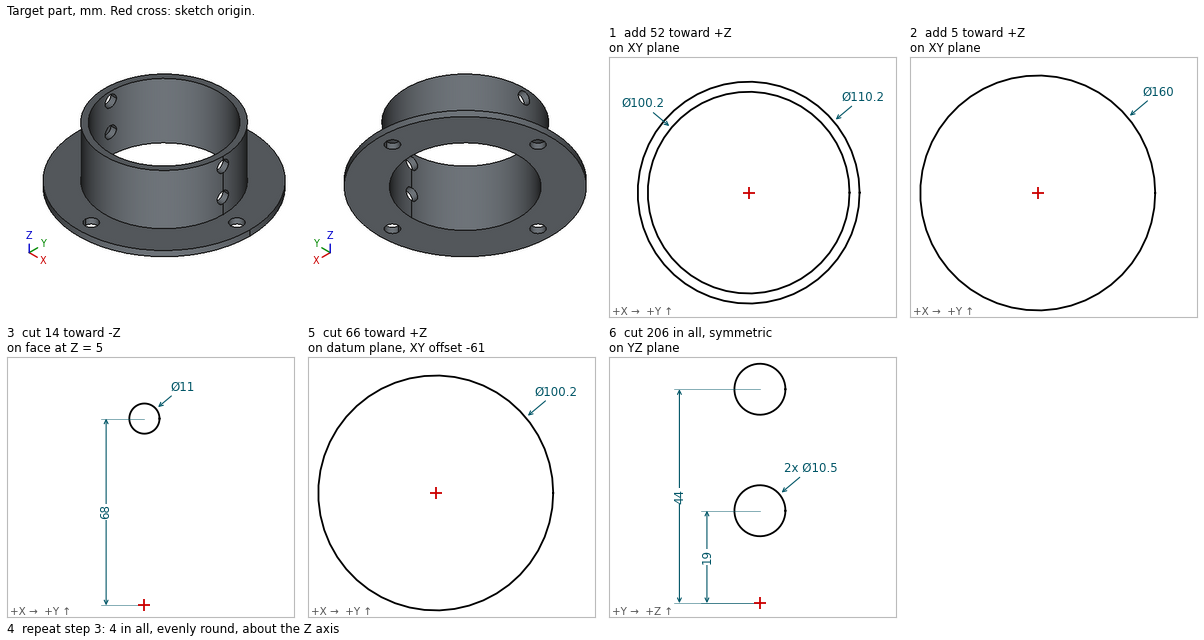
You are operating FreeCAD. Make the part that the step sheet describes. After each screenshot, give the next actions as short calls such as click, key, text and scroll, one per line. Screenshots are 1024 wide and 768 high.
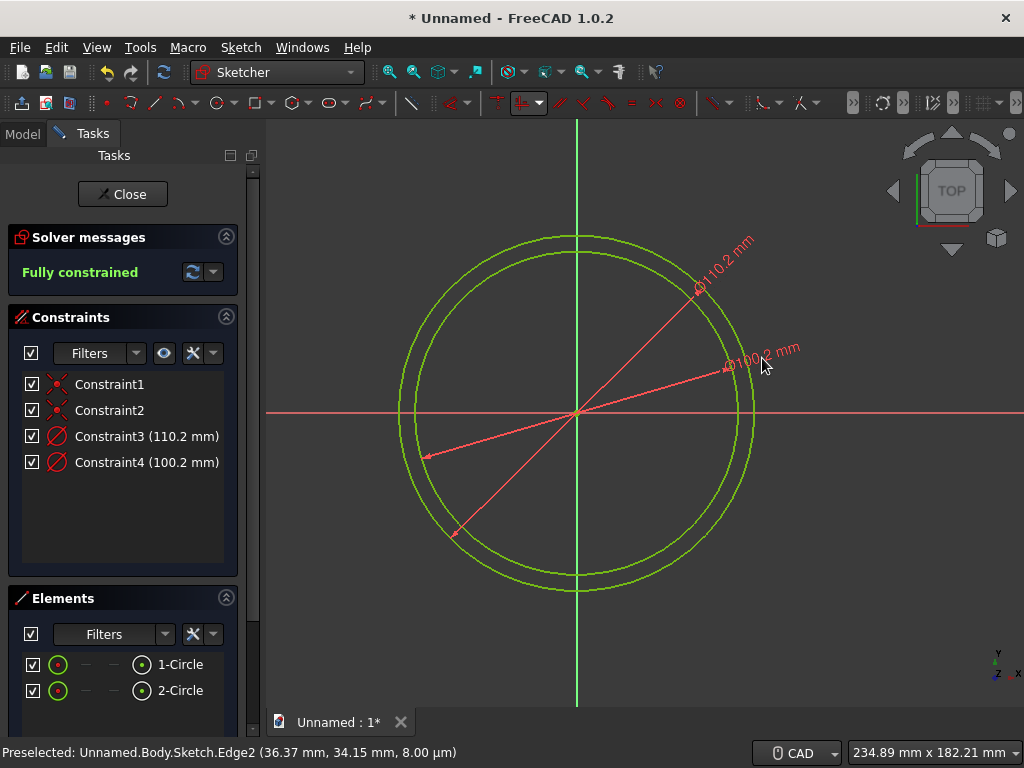
click(123, 194)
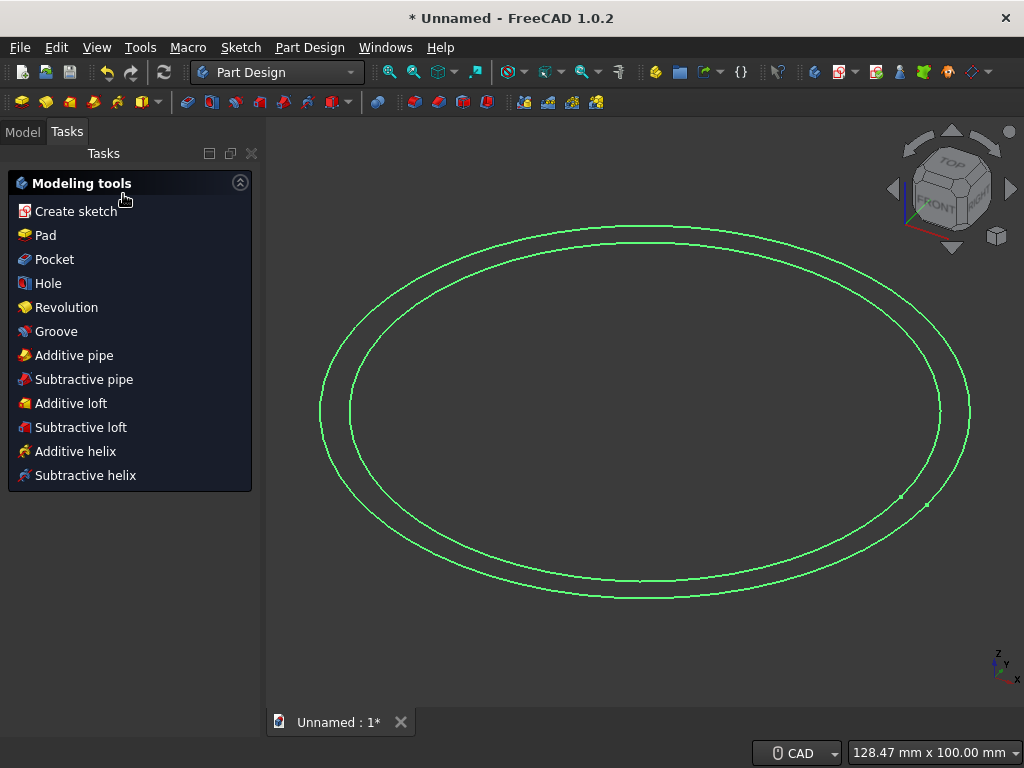
click(22, 102)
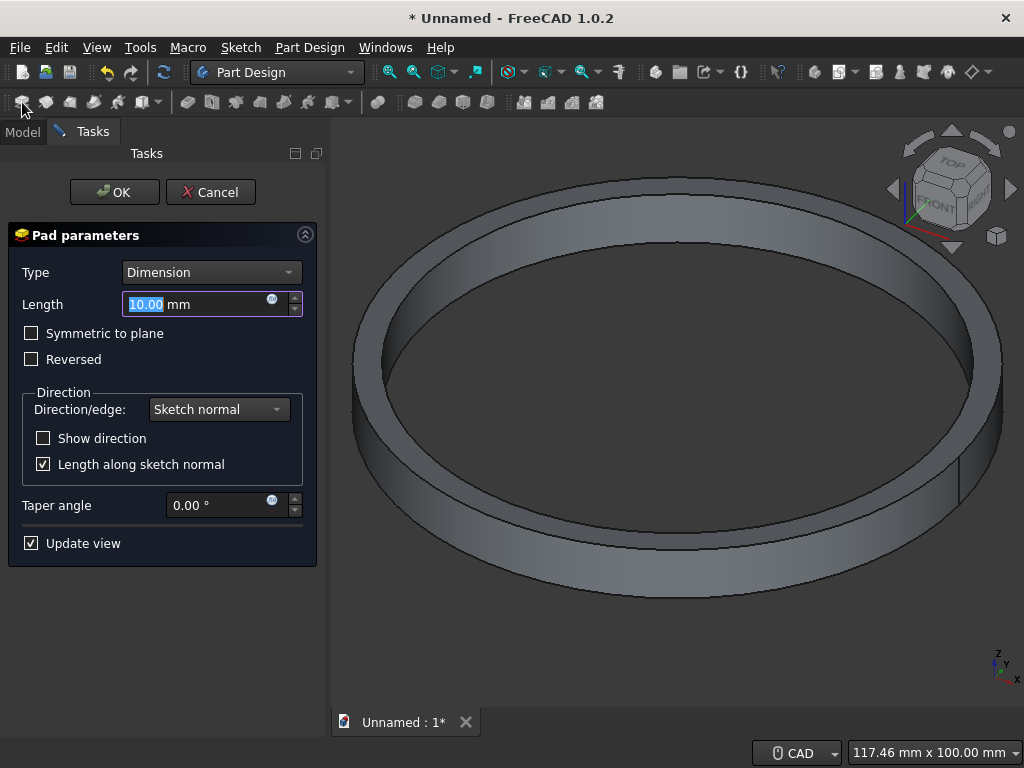
text(52)
key(Tab)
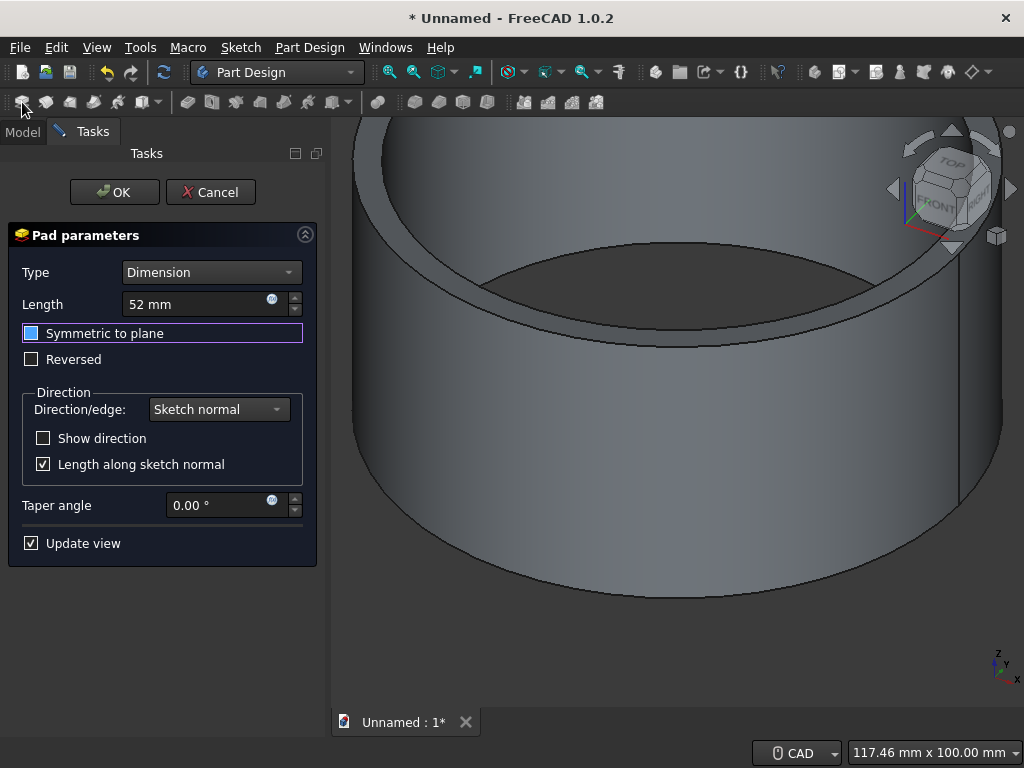
click(115, 192)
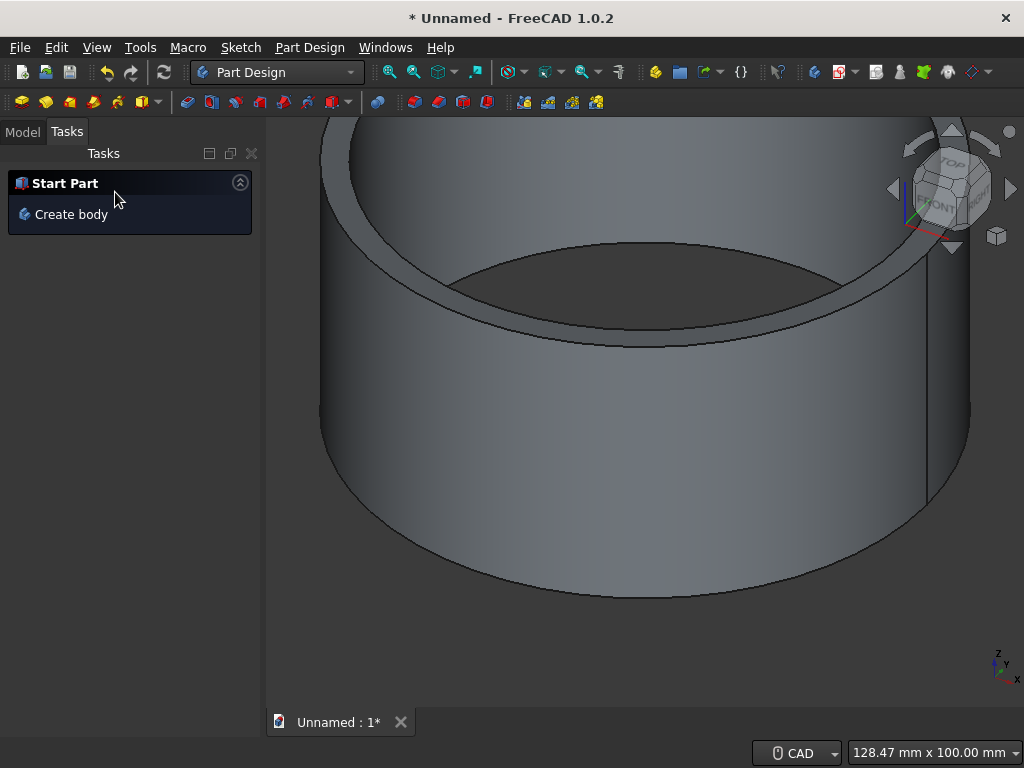
click(390, 72)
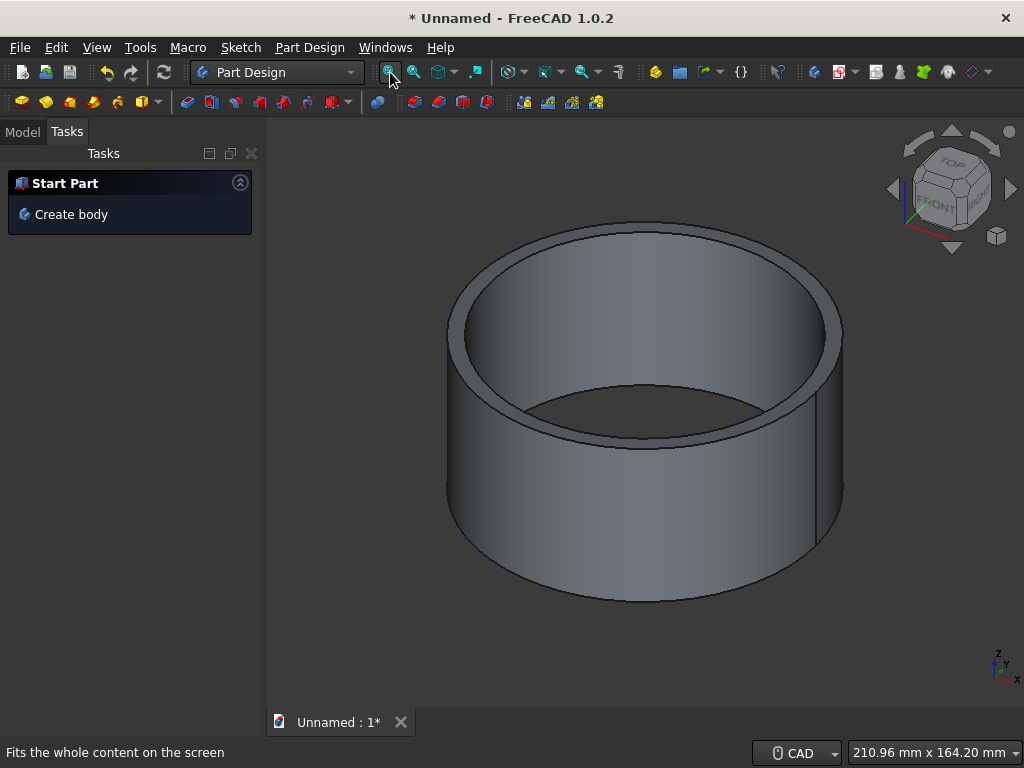
click(840, 72)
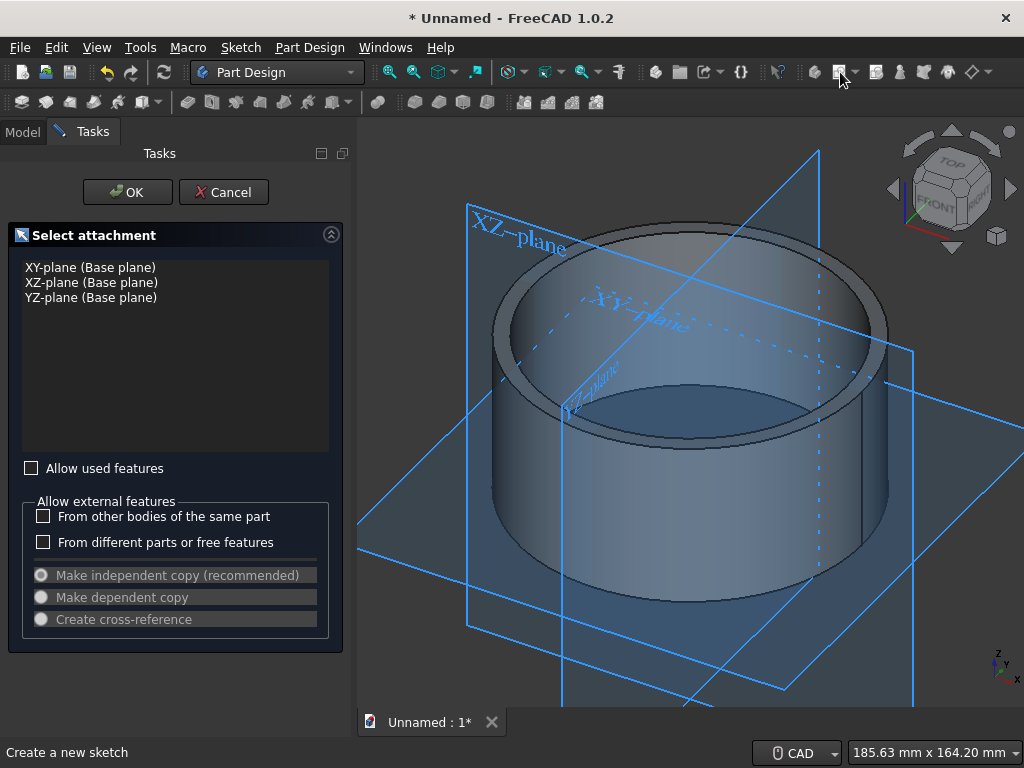
click(82, 268)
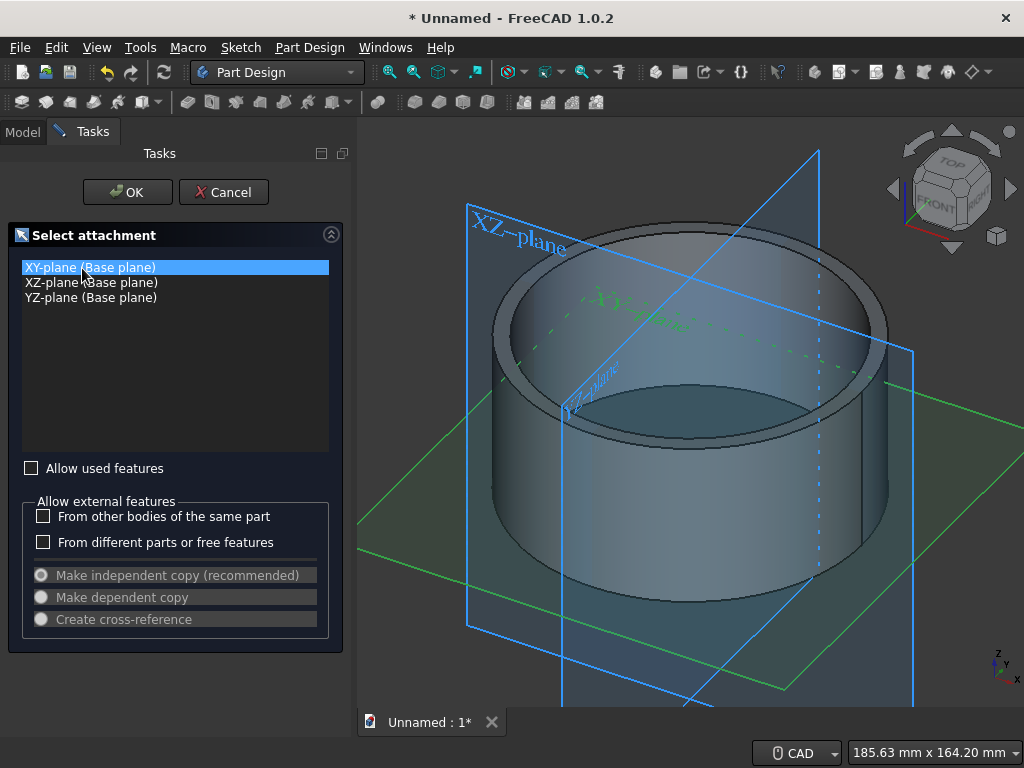
click(128, 192)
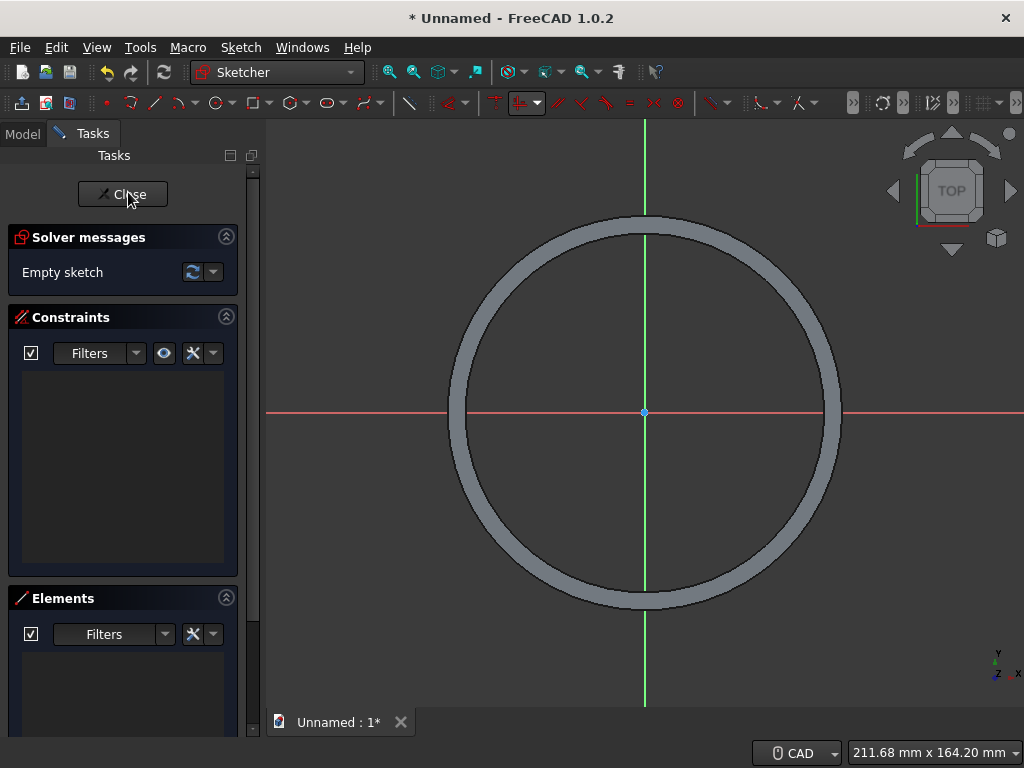
click(70, 104)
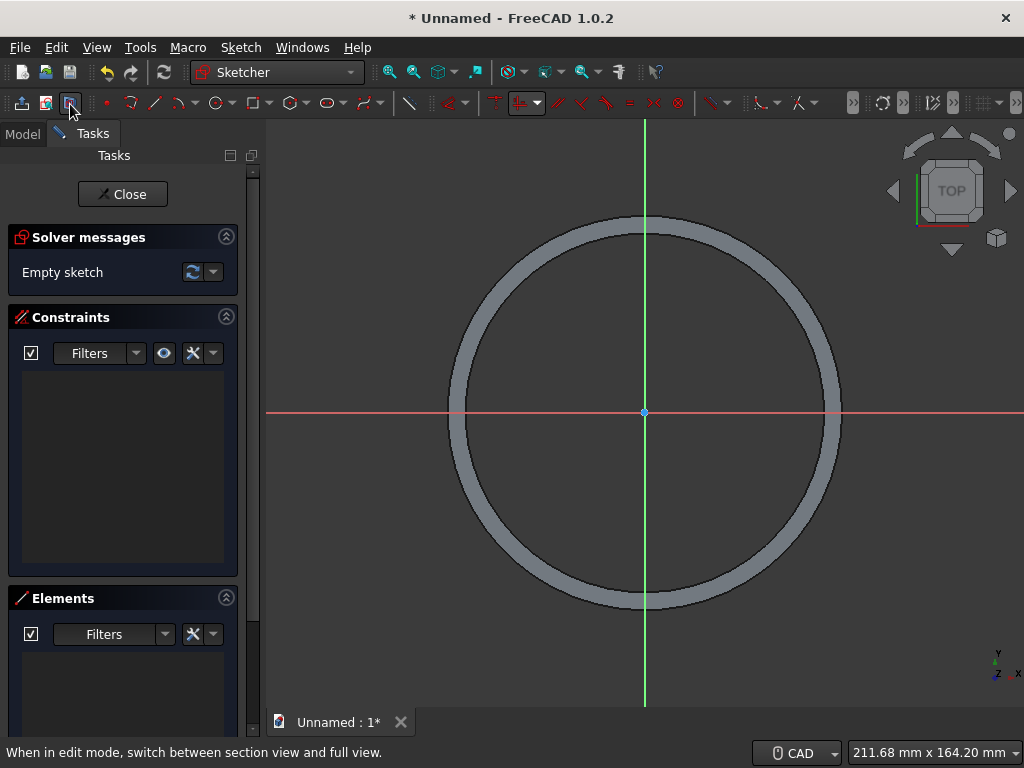
scroll(438, 413, down, 2)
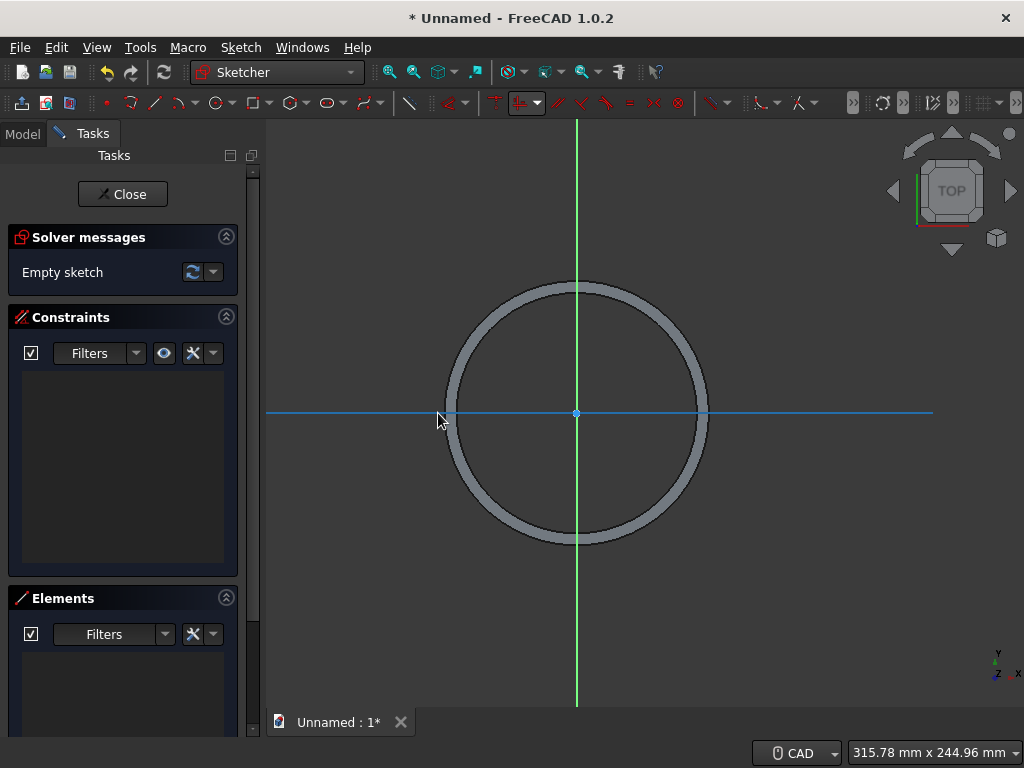
click(216, 104)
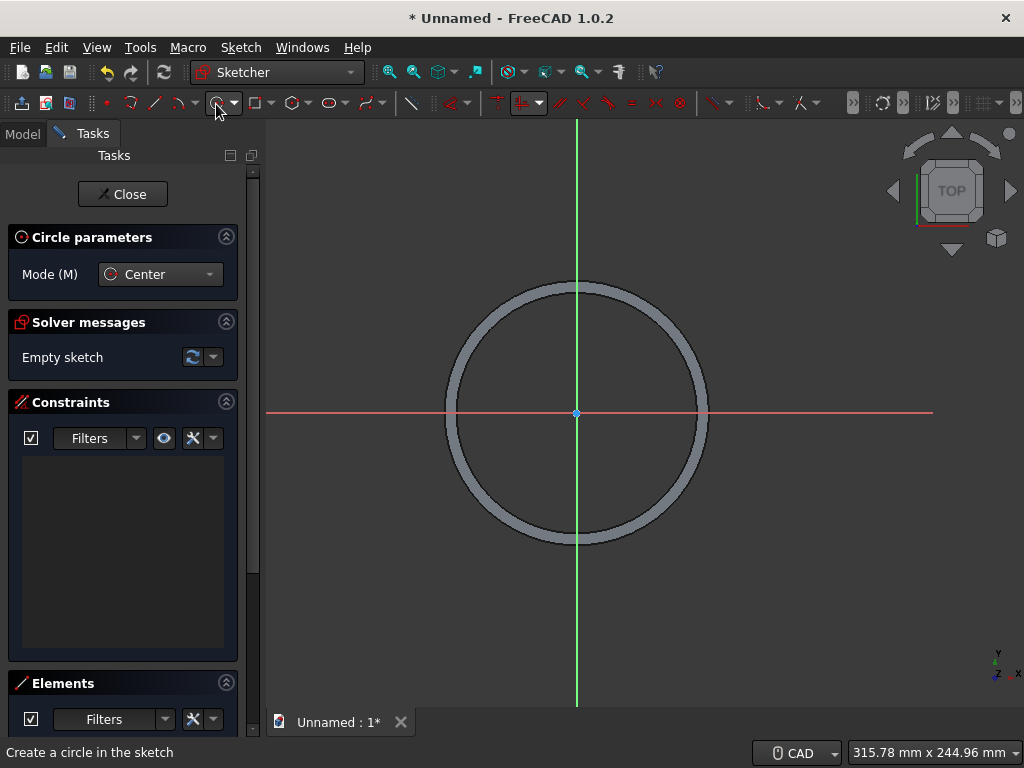
click(577, 413)
click(713, 277)
key(Escape)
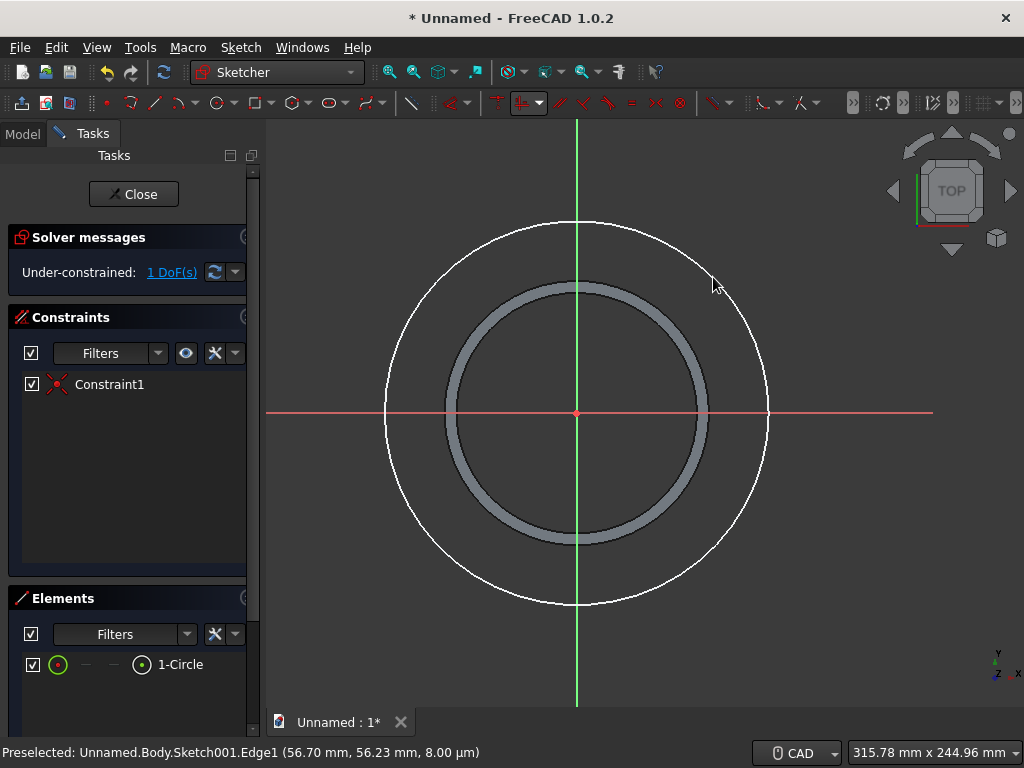
click(450, 104)